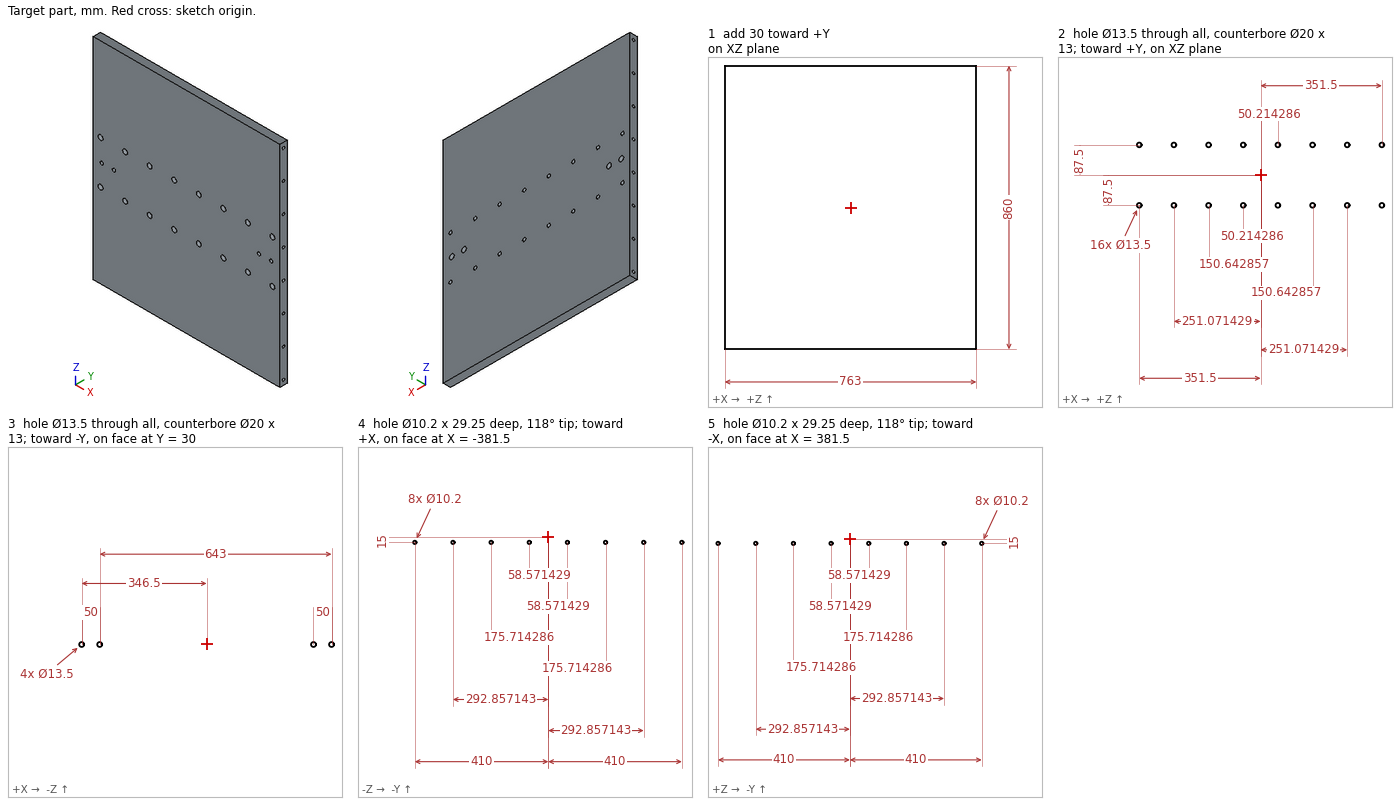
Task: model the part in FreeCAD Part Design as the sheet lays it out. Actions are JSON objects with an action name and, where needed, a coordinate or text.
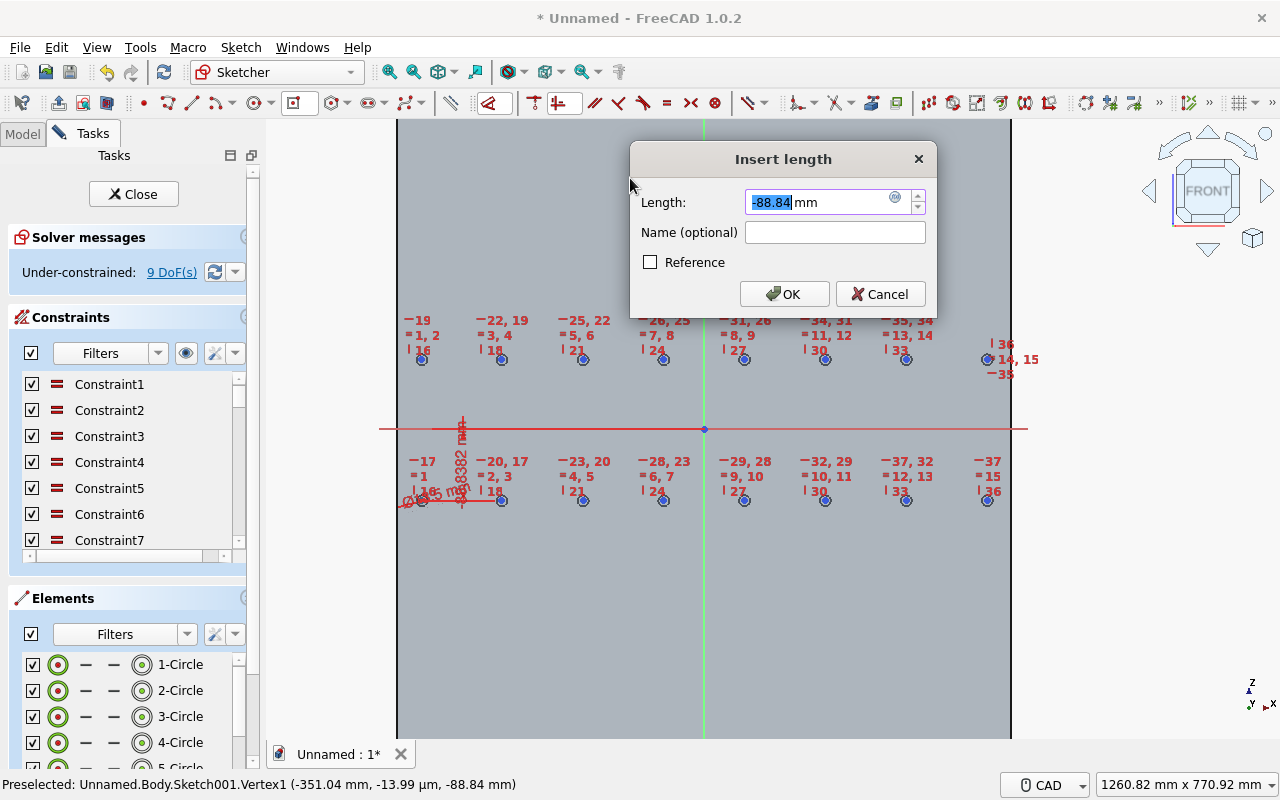
{"action": "type", "text": "-87.5"}
{"action": "key", "text": "Return"}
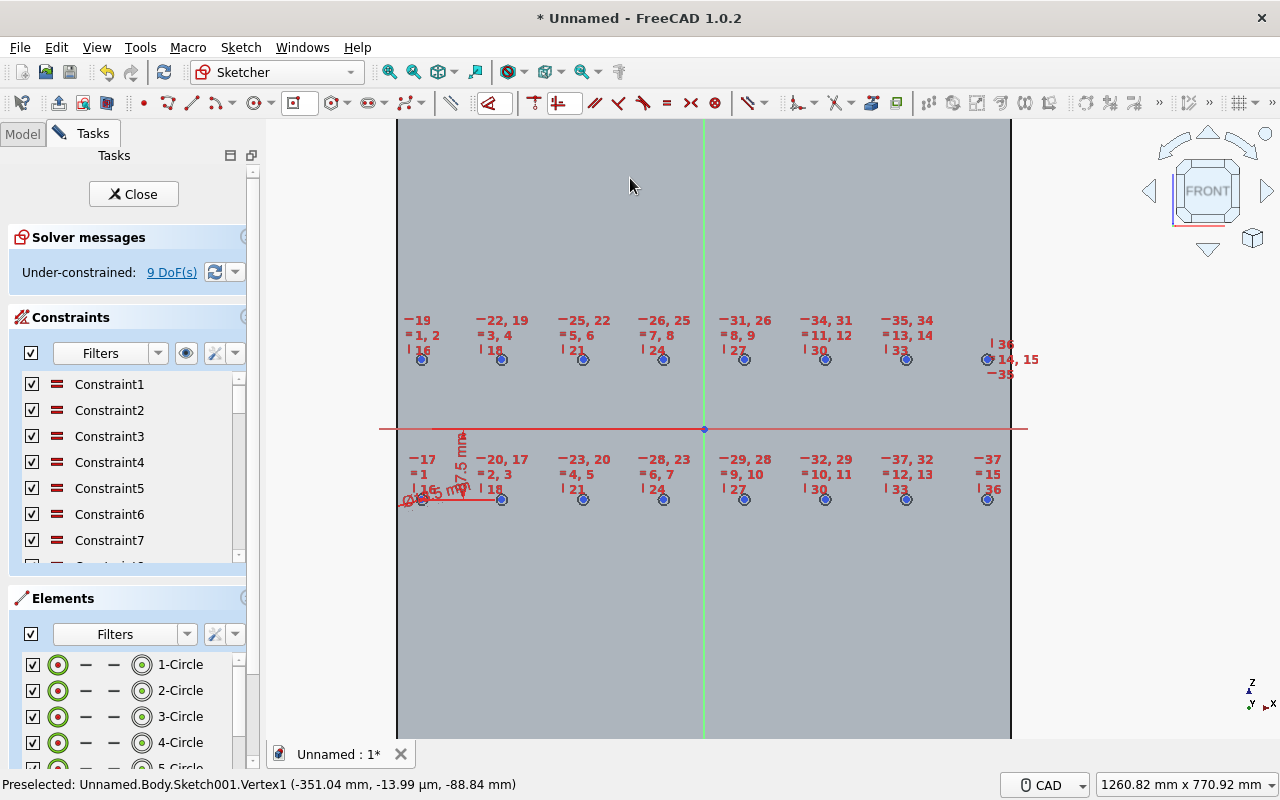
{"action": "left_click", "coordinate": [422, 360]}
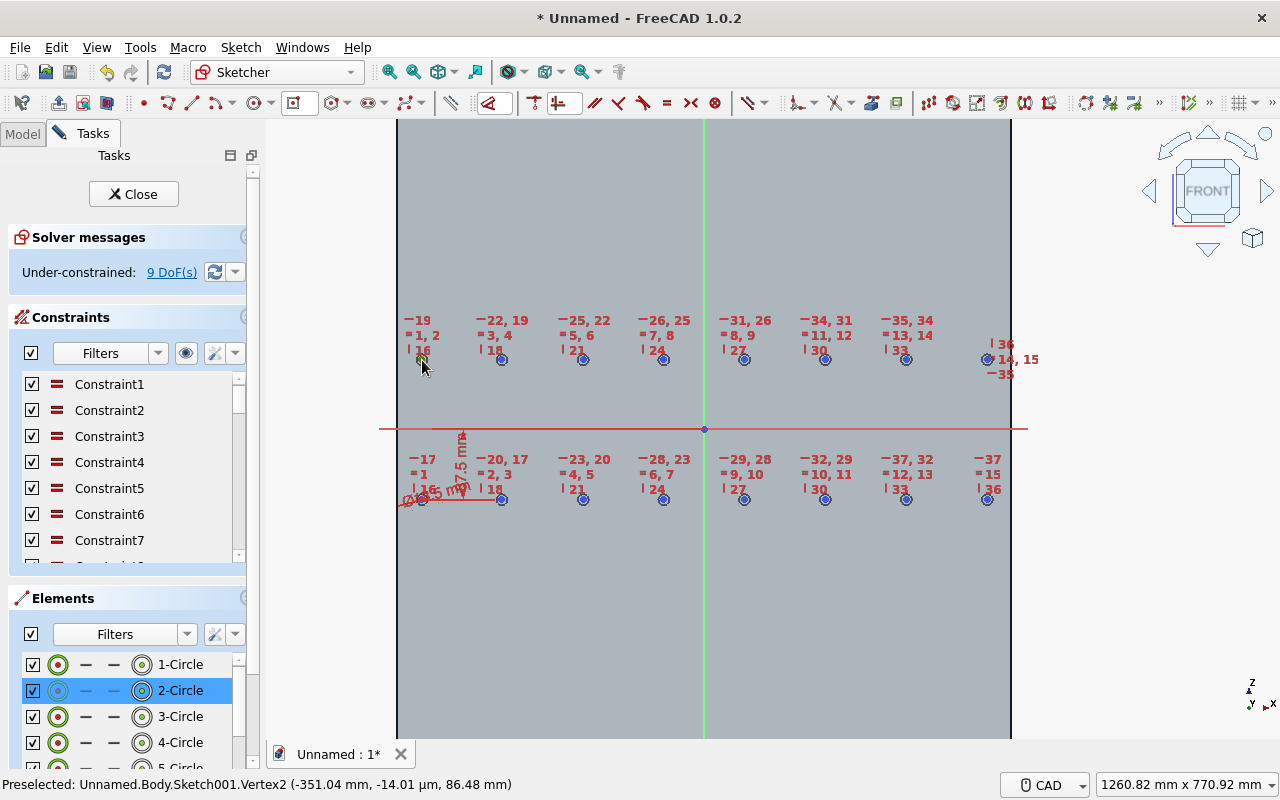
{"action": "left_click", "coordinate": [506, 104]}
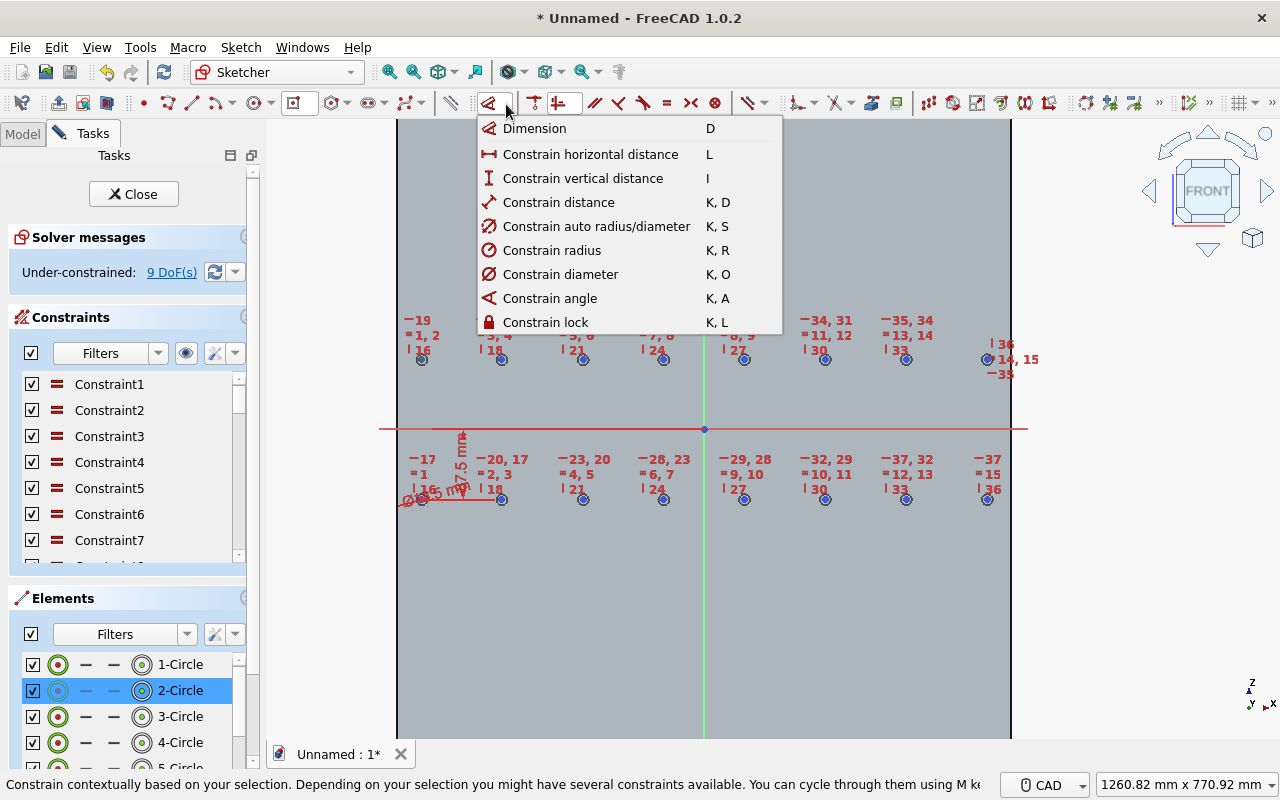
{"action": "left_click", "coordinate": [630, 178]}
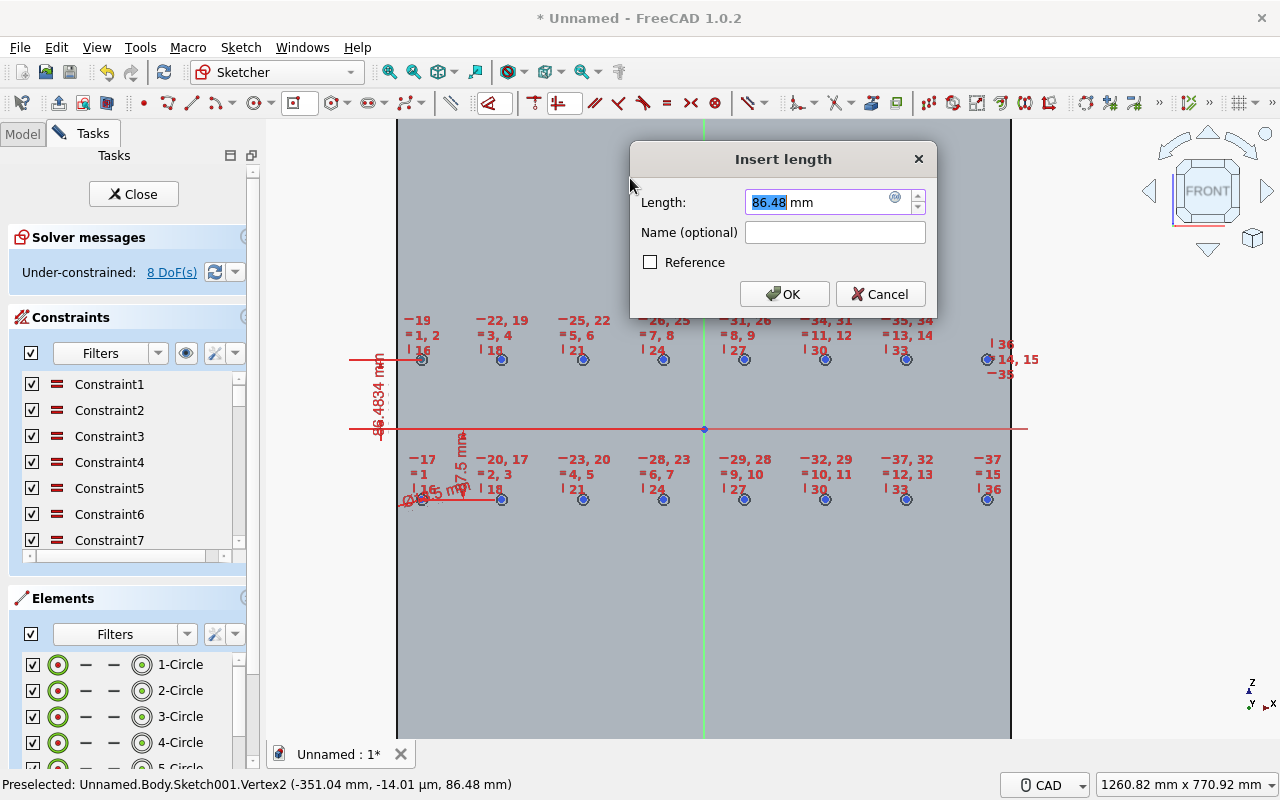
{"action": "type", "text": "87.5"}
{"action": "key", "text": "Return"}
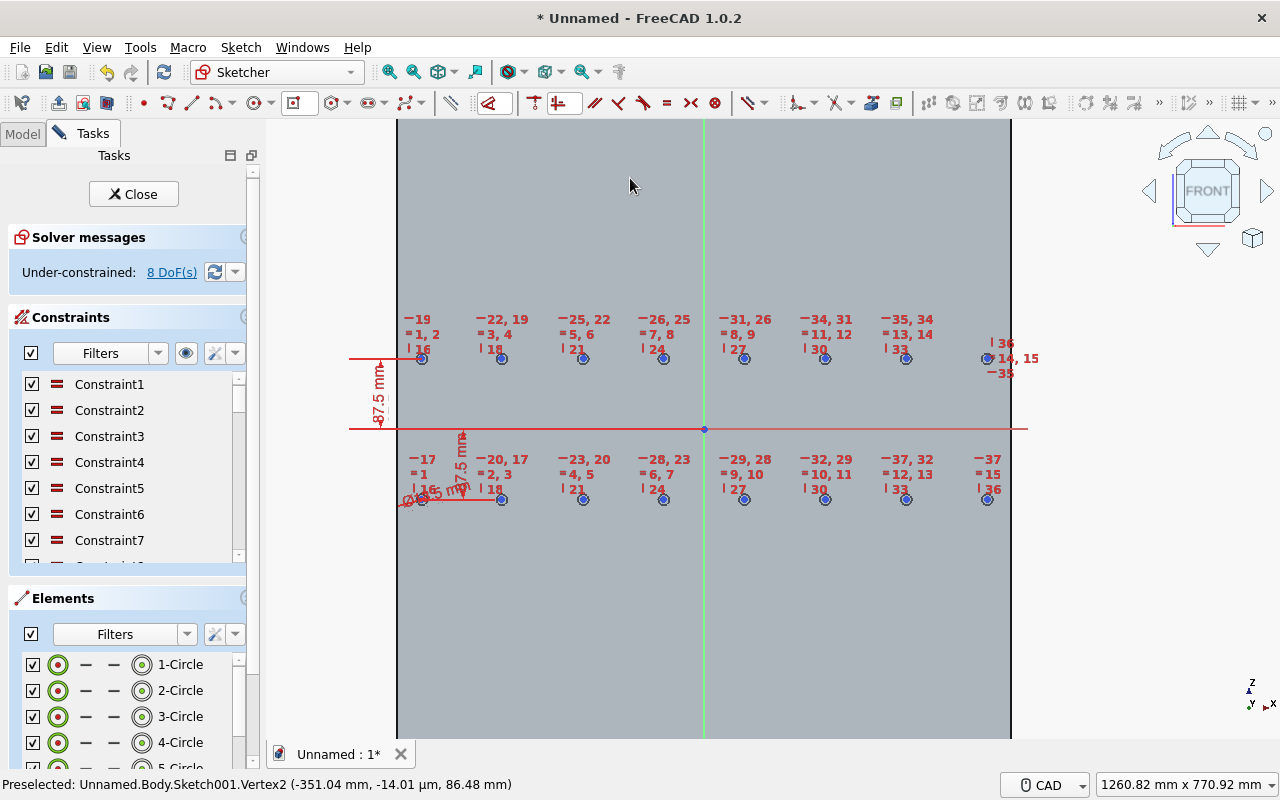
{"action": "left_click", "coordinate": [422, 500]}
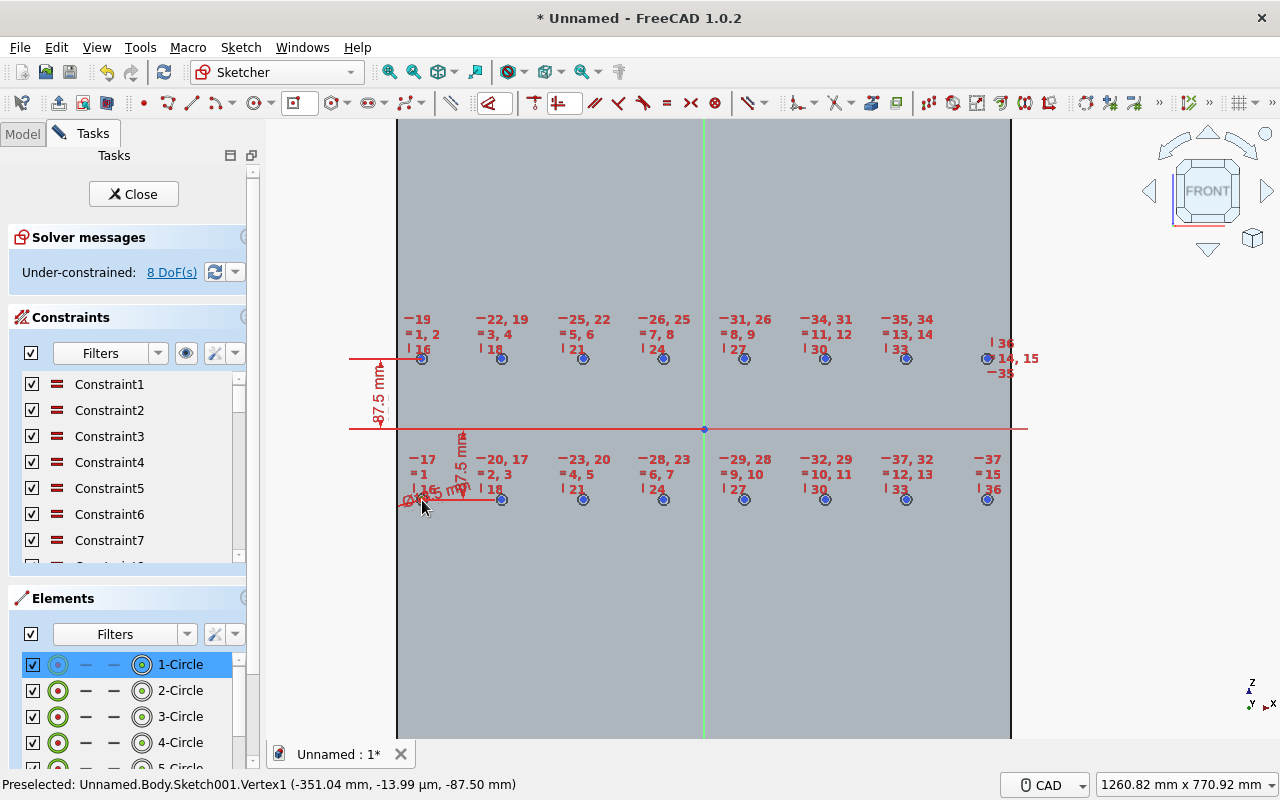
{"action": "key", "text": "l"}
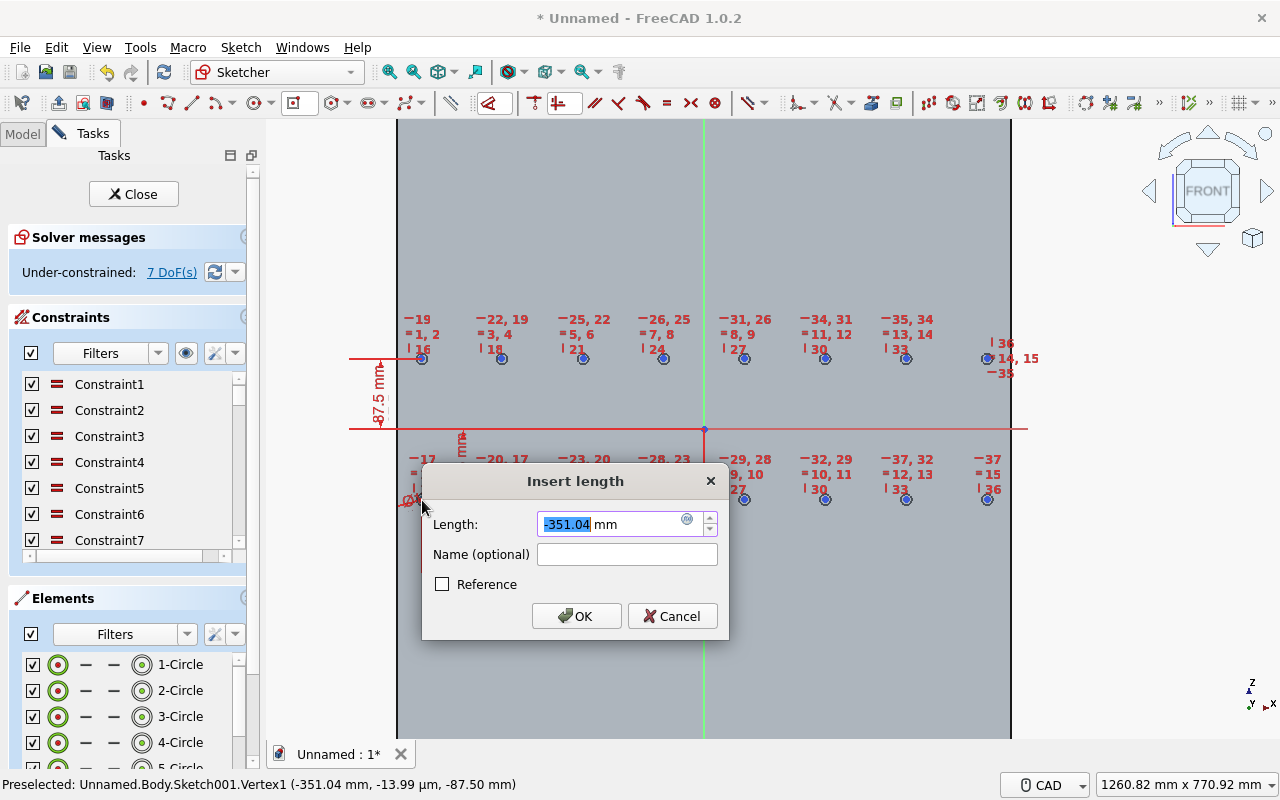
{"action": "type", "text": "-351.5"}
{"action": "key", "text": "Return"}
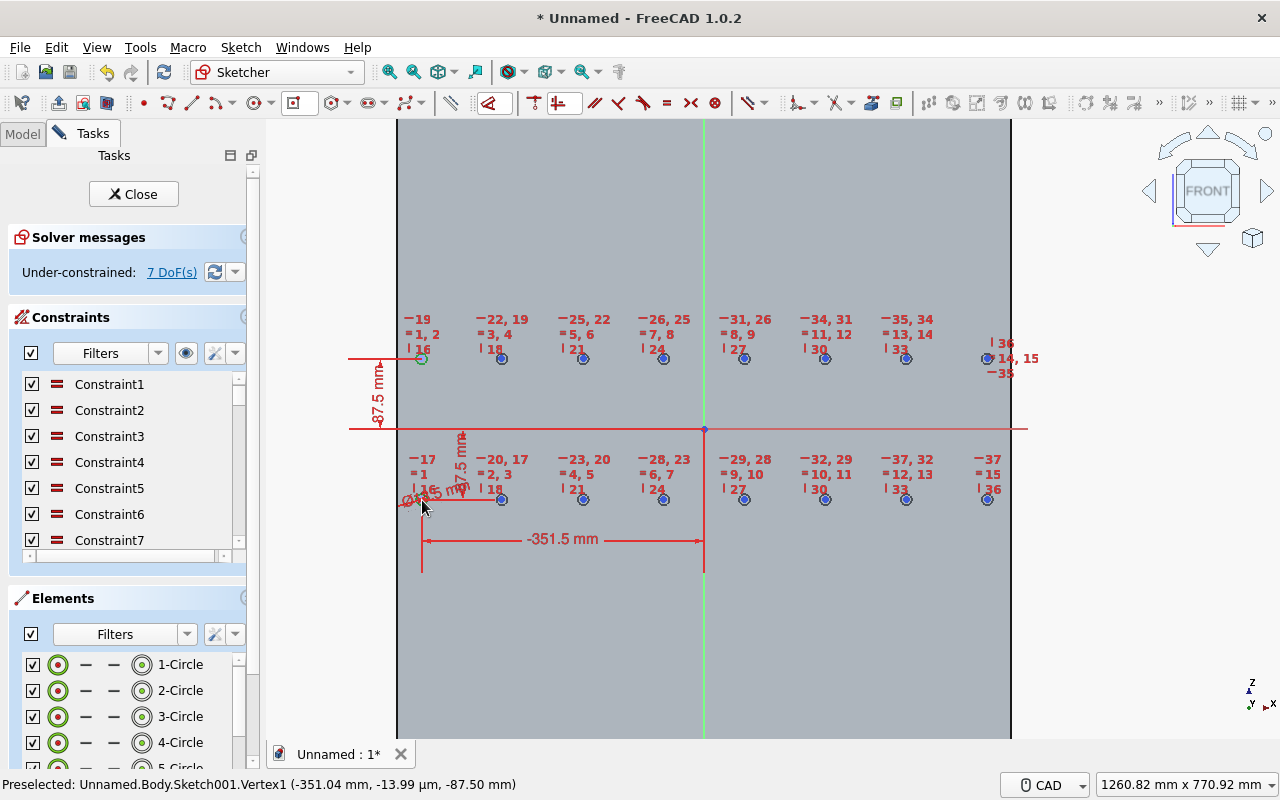
{"action": "left_click", "coordinate": [987, 359]}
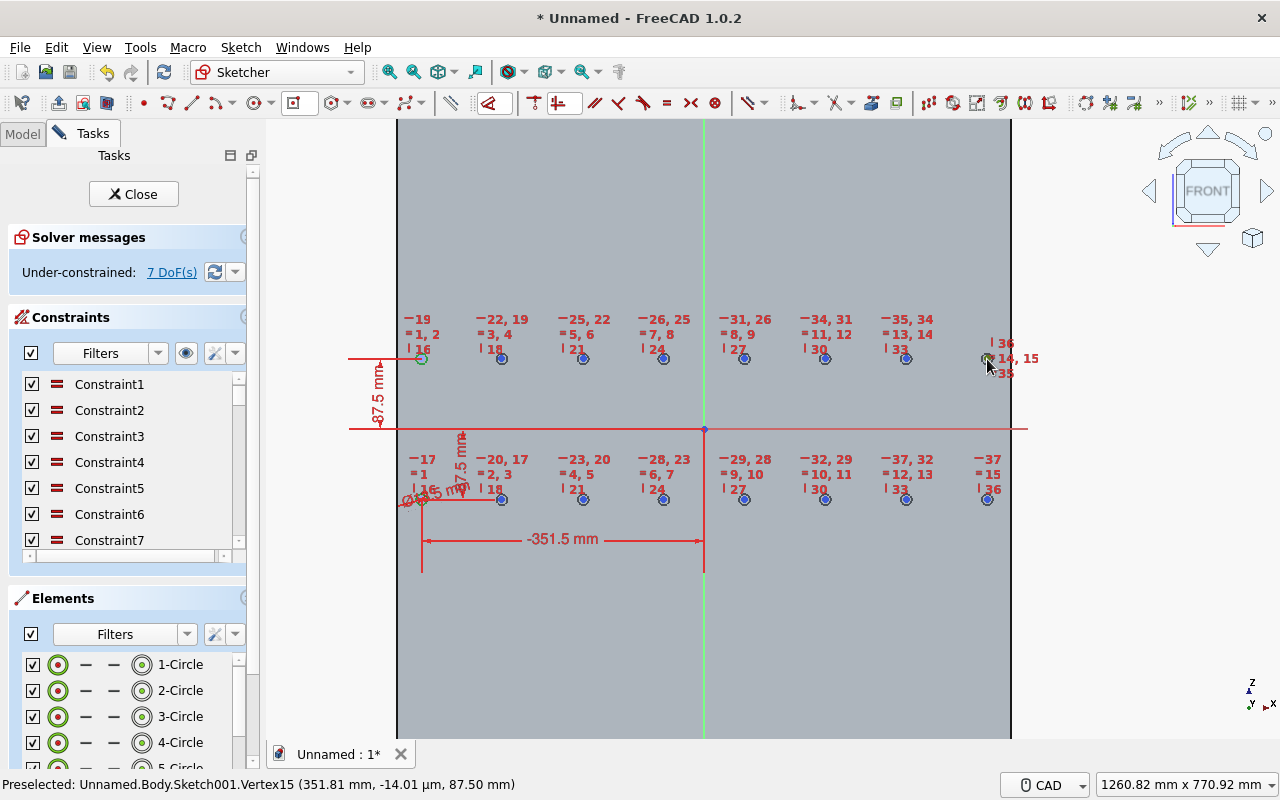
{"action": "key", "text": "l"}